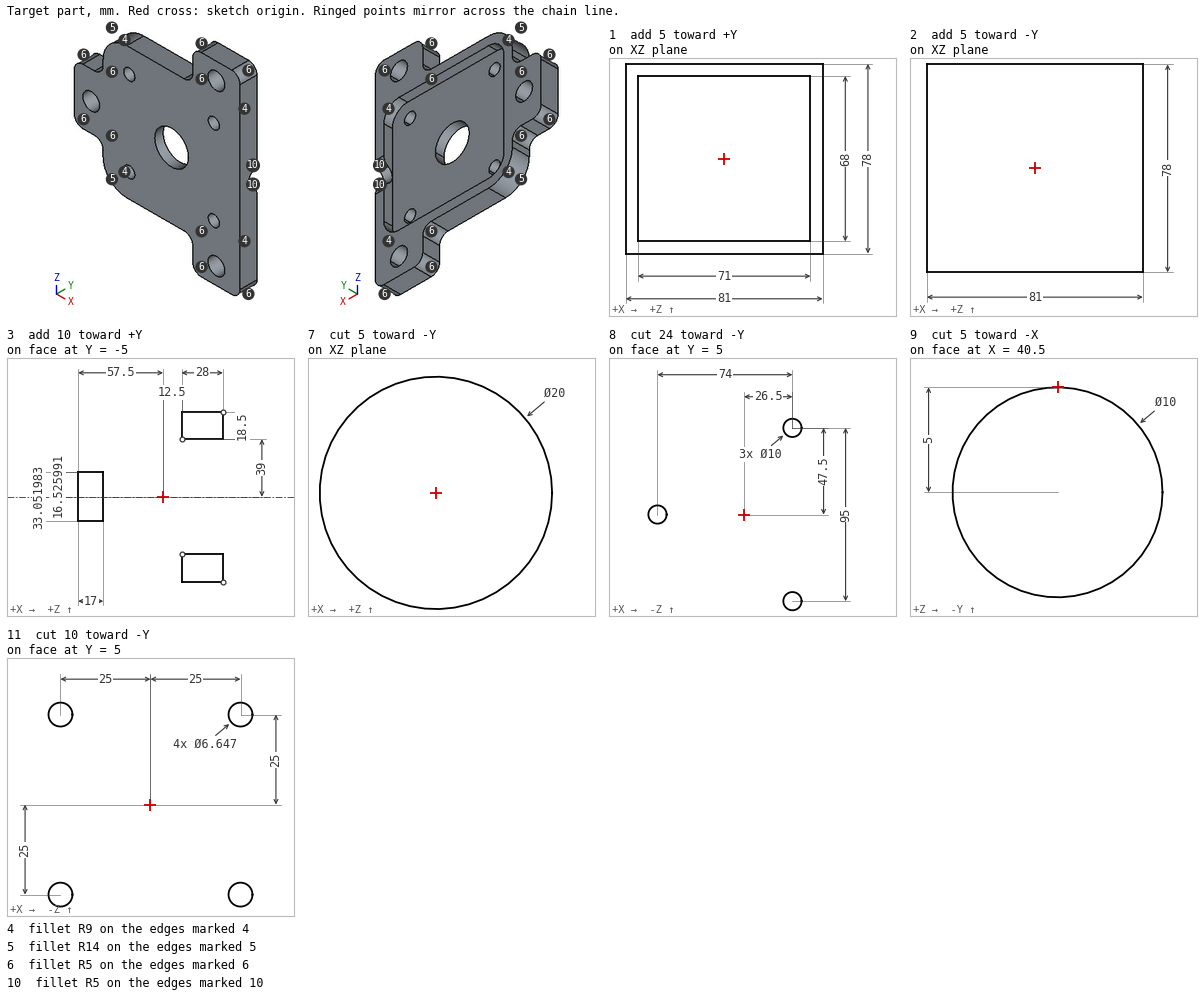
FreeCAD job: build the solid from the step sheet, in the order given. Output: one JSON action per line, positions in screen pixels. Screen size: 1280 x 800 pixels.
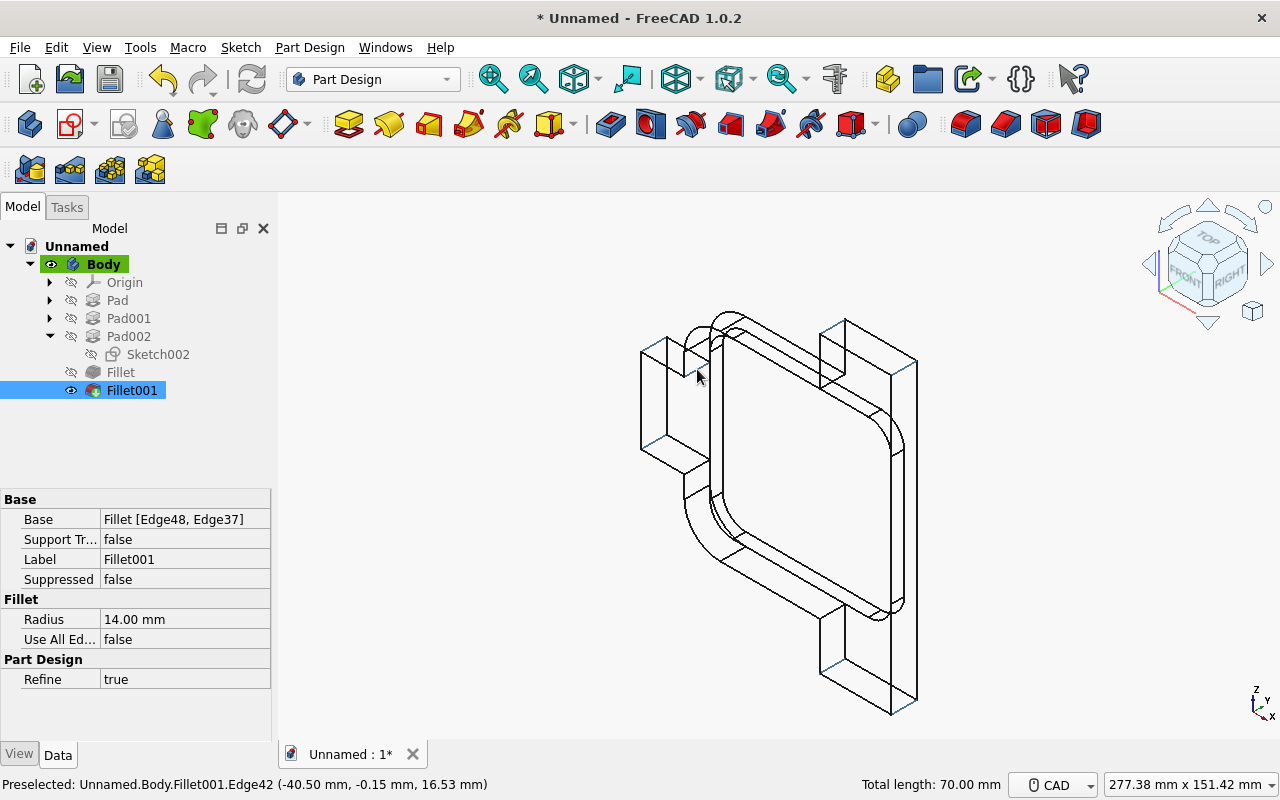
{"action": "left_click", "coordinate": [697, 466], "text": "ctrl"}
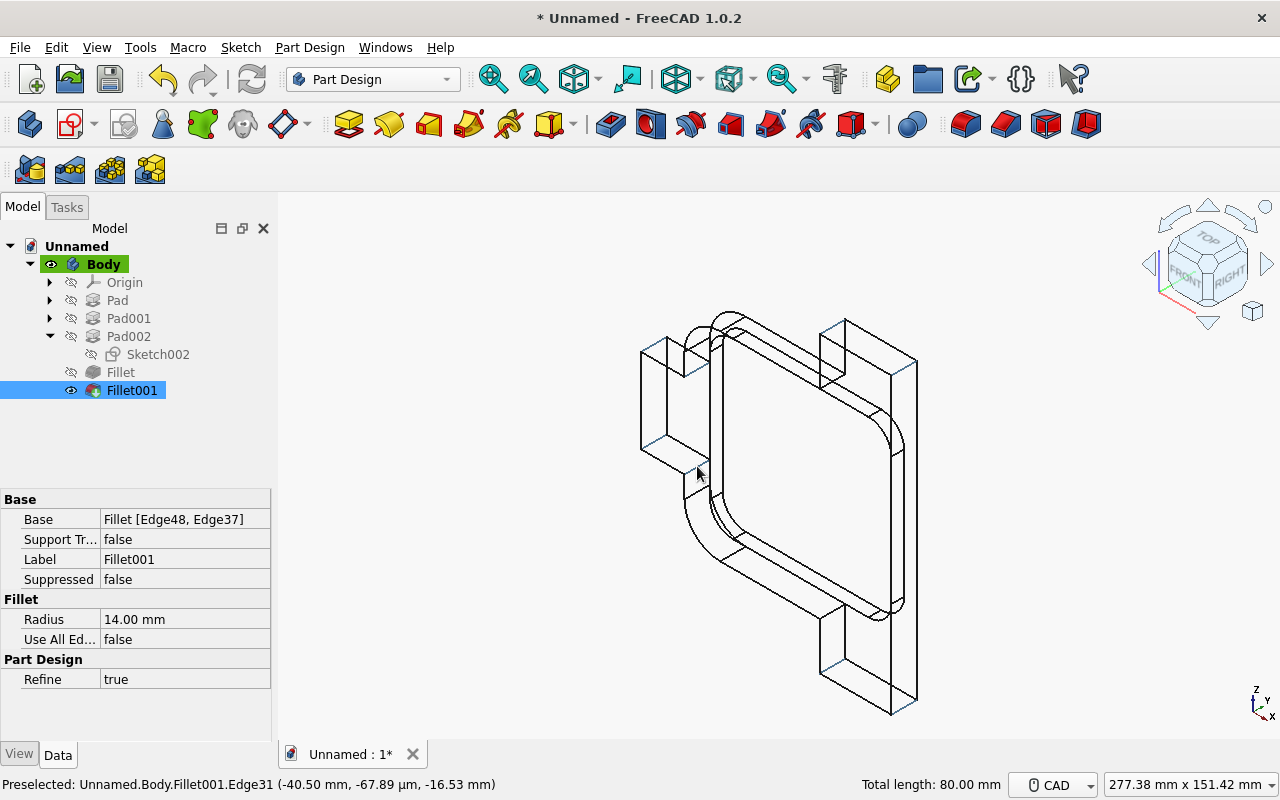
{"action": "left_click", "coordinate": [833, 611], "text": "ctrl"}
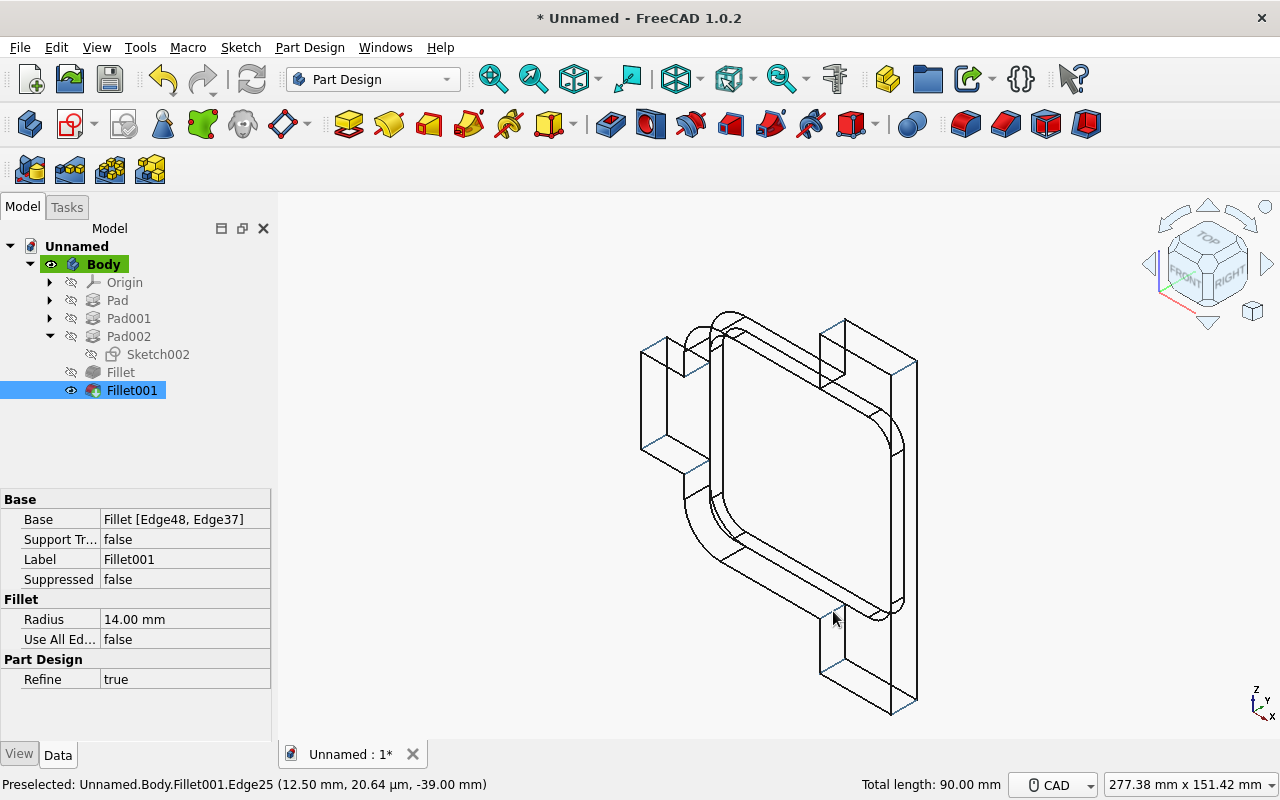
{"action": "left_click", "coordinate": [833, 380], "text": "ctrl"}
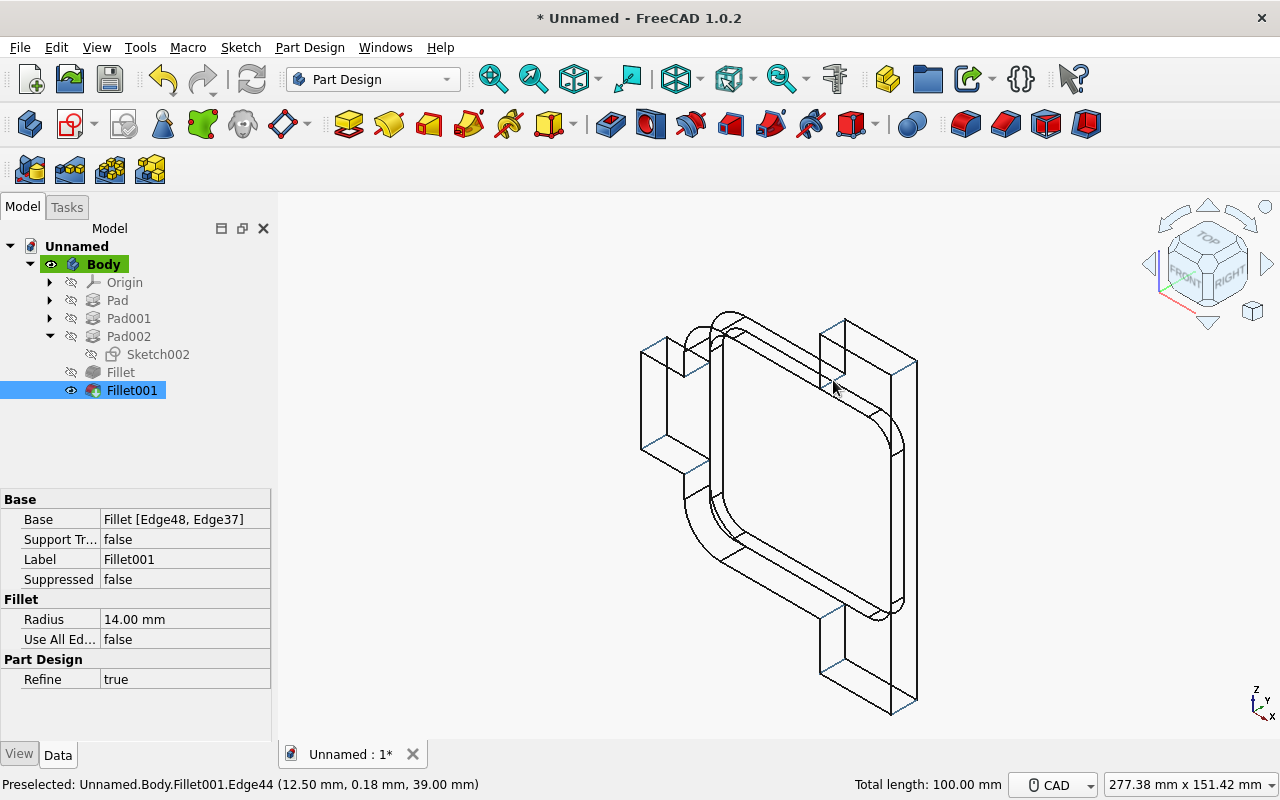
{"action": "key", "text": "v 1"}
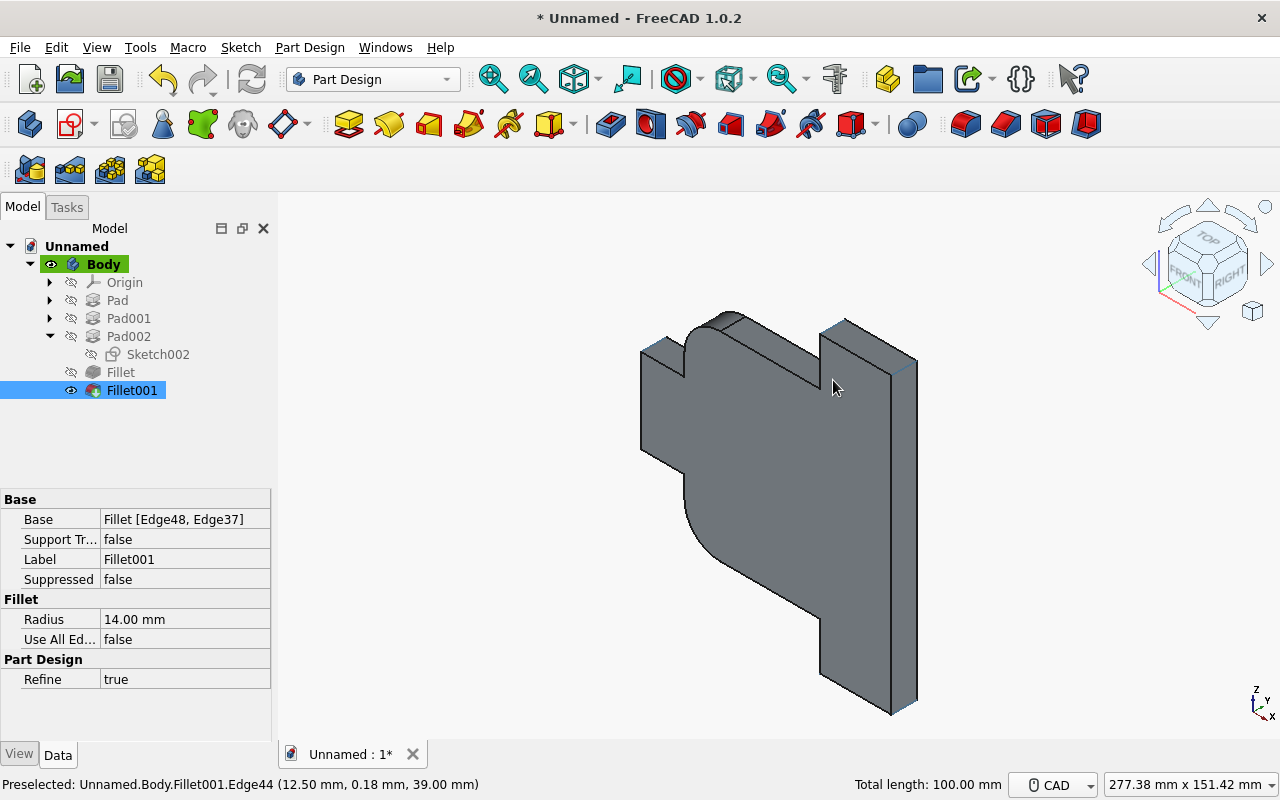
{"action": "left_click", "coordinate": [966, 124]}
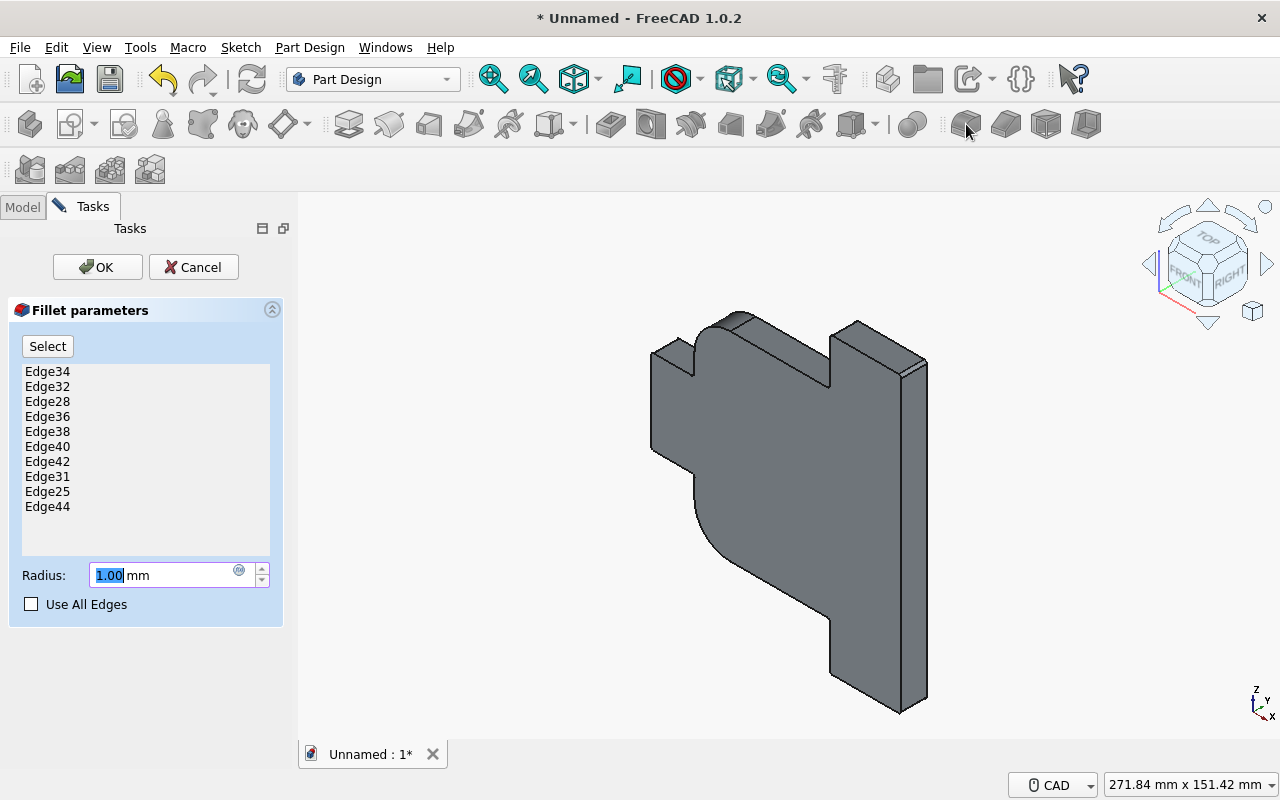
{"action": "type", "text": "5"}
{"action": "key", "text": "Tab"}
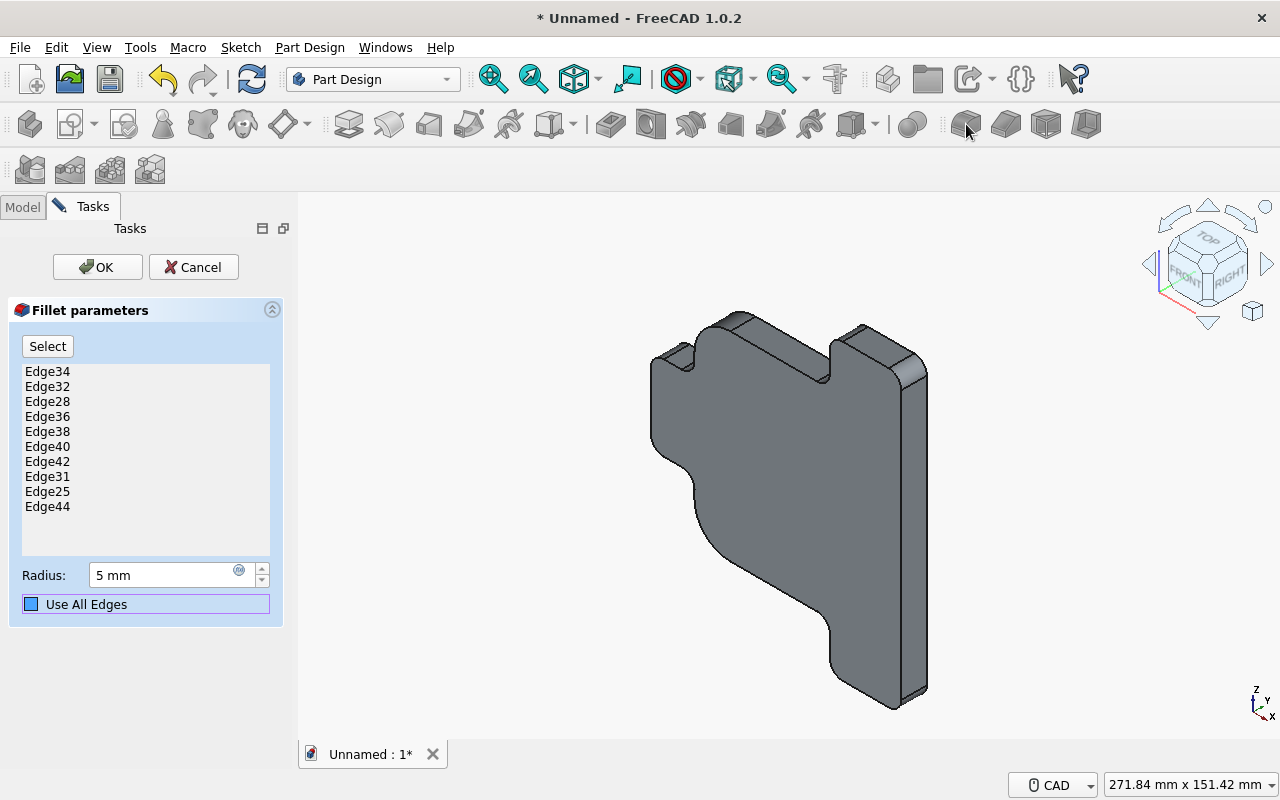
{"action": "left_click", "coordinate": [98, 267]}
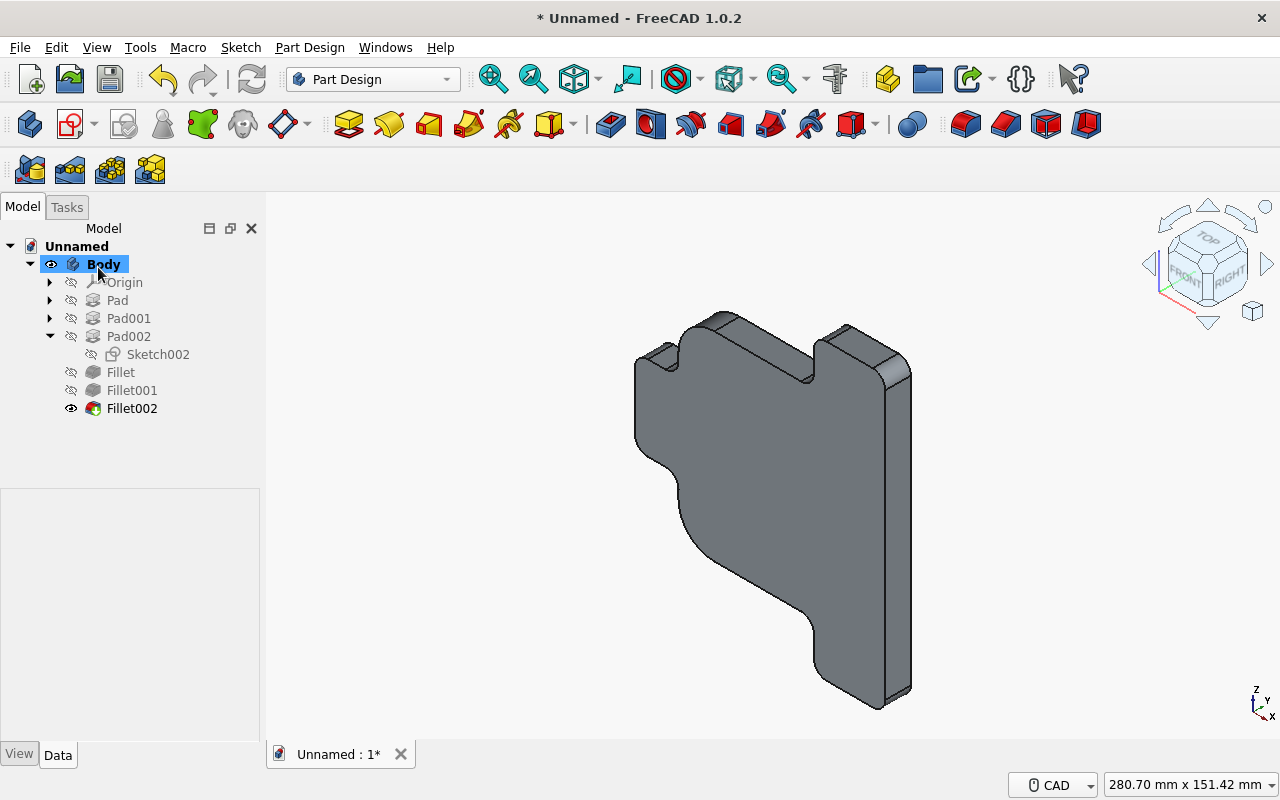
{"action": "left_click", "coordinate": [70, 124]}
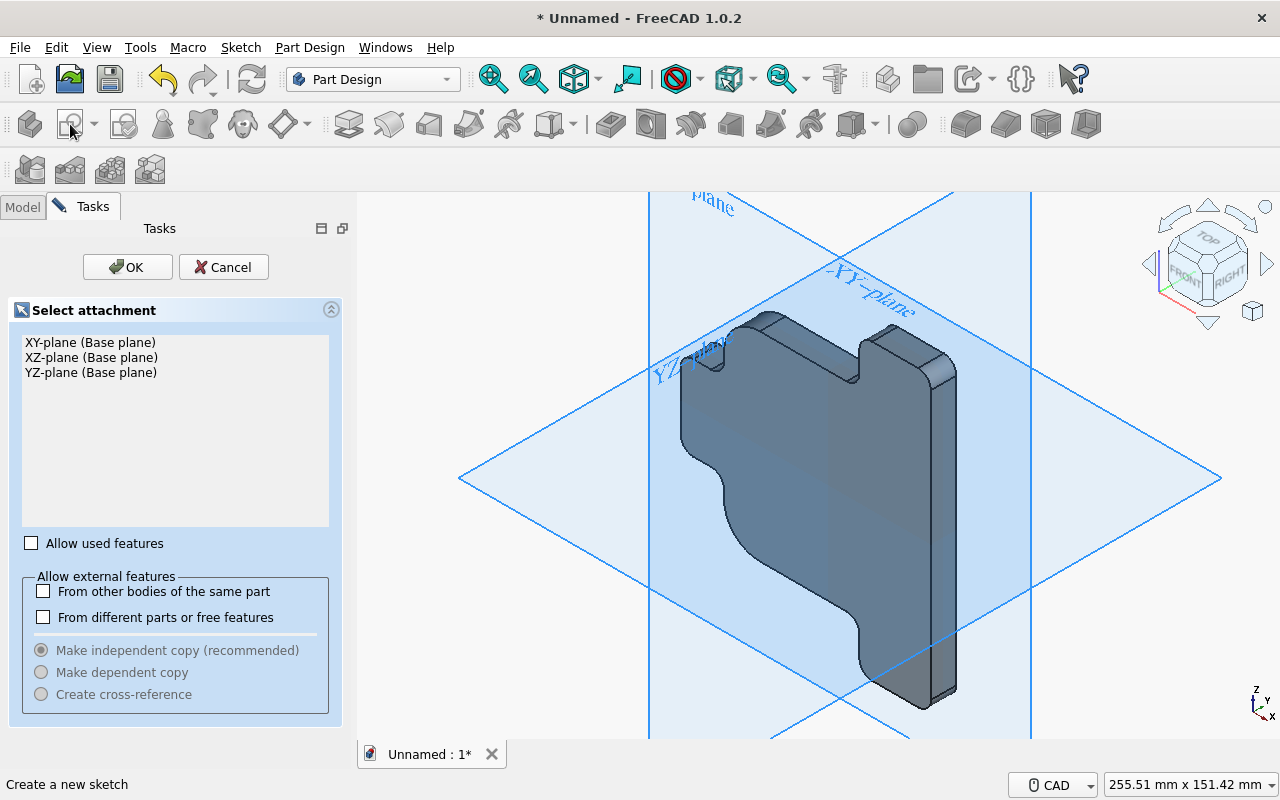
{"action": "left_click", "coordinate": [82, 358]}